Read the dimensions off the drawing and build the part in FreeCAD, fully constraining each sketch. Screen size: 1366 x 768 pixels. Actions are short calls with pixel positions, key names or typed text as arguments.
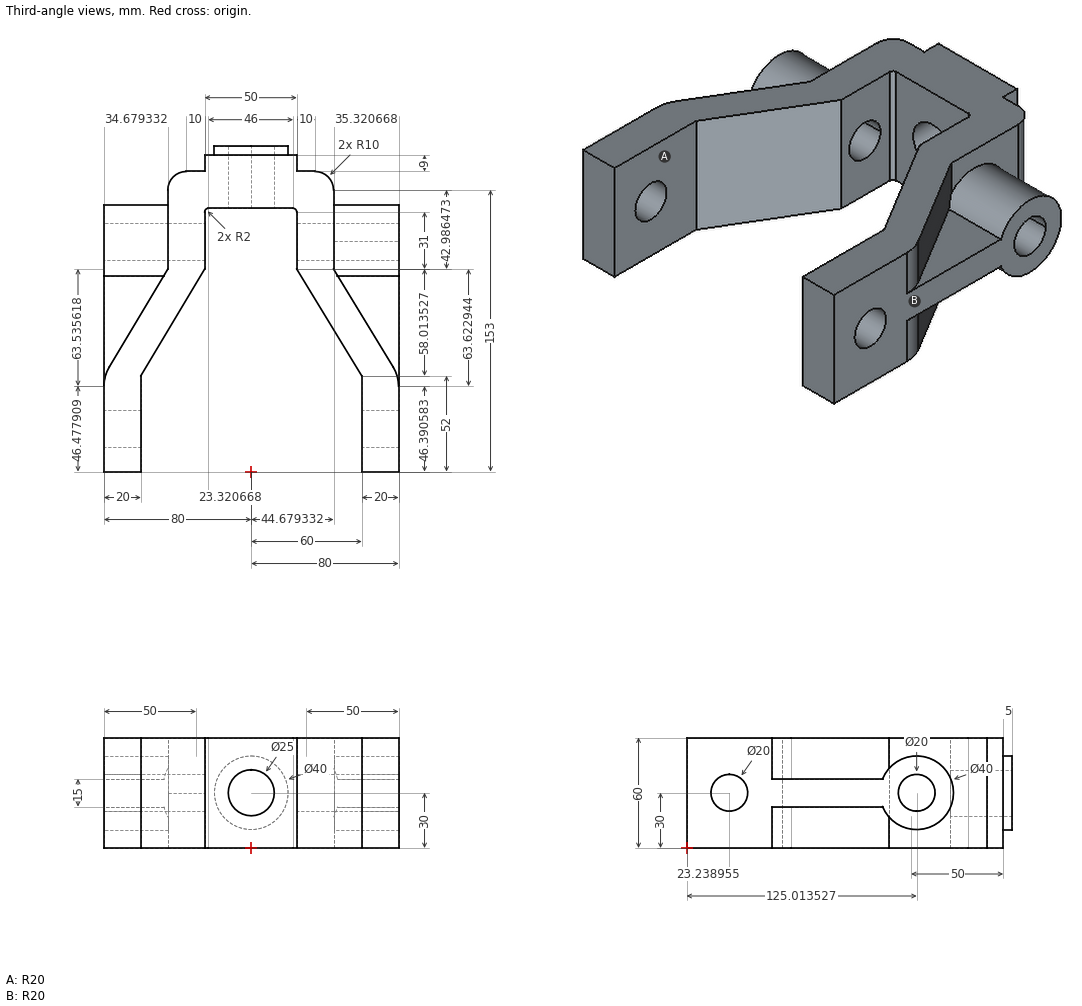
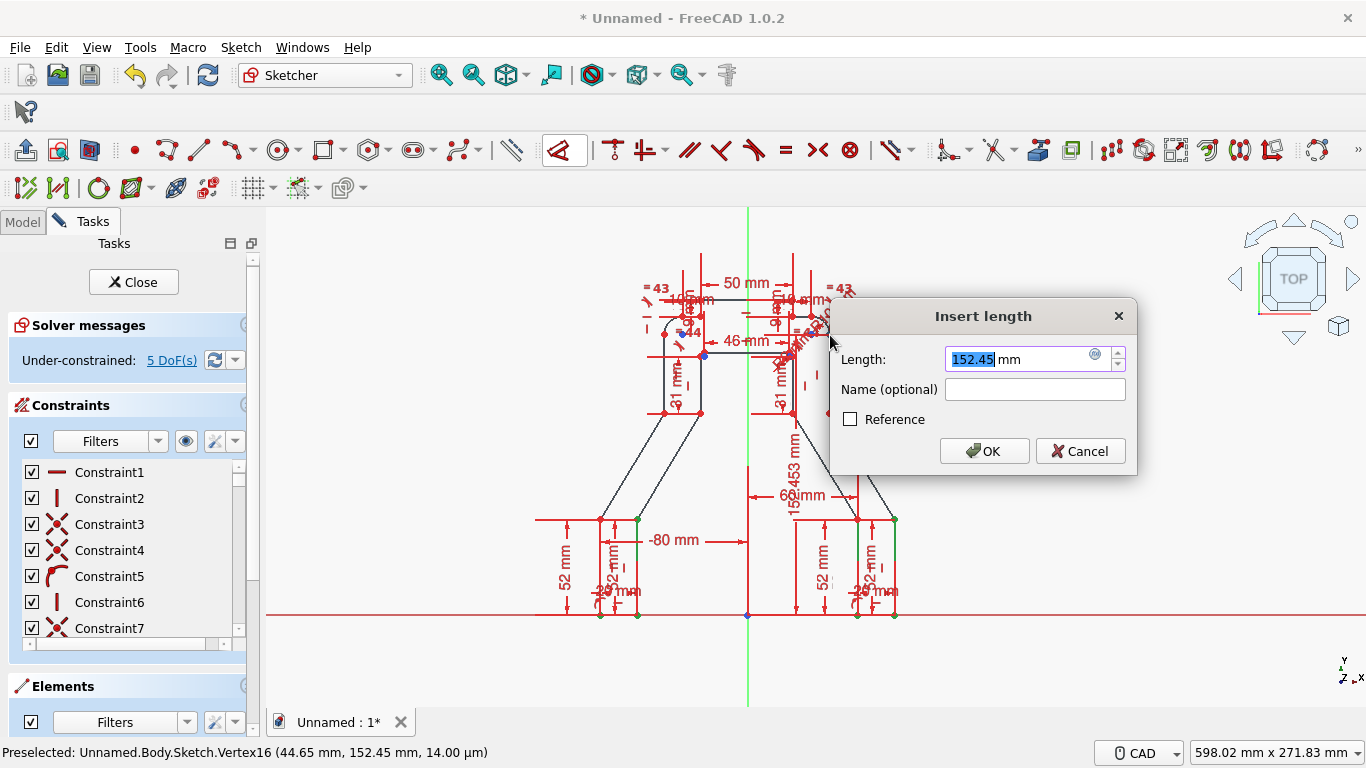
text(153)
key(Return)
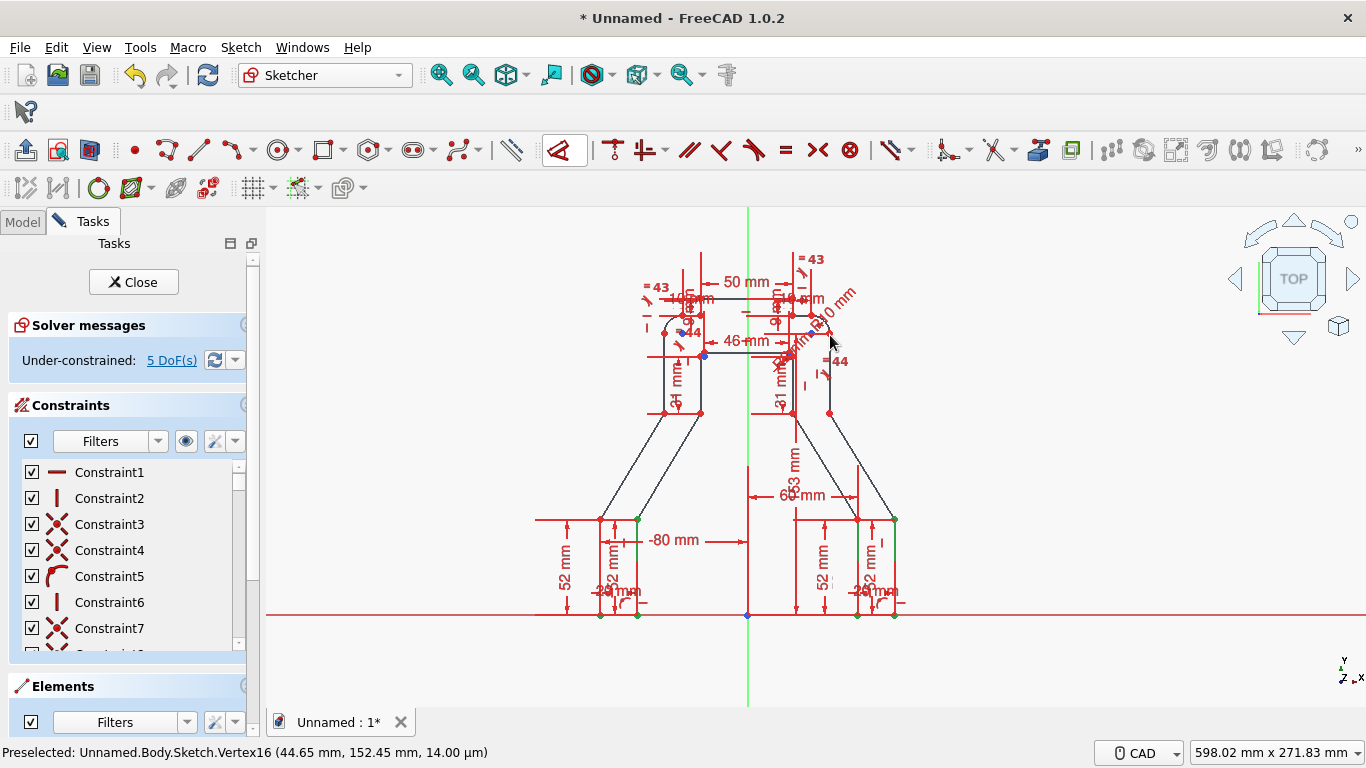
click(830, 390)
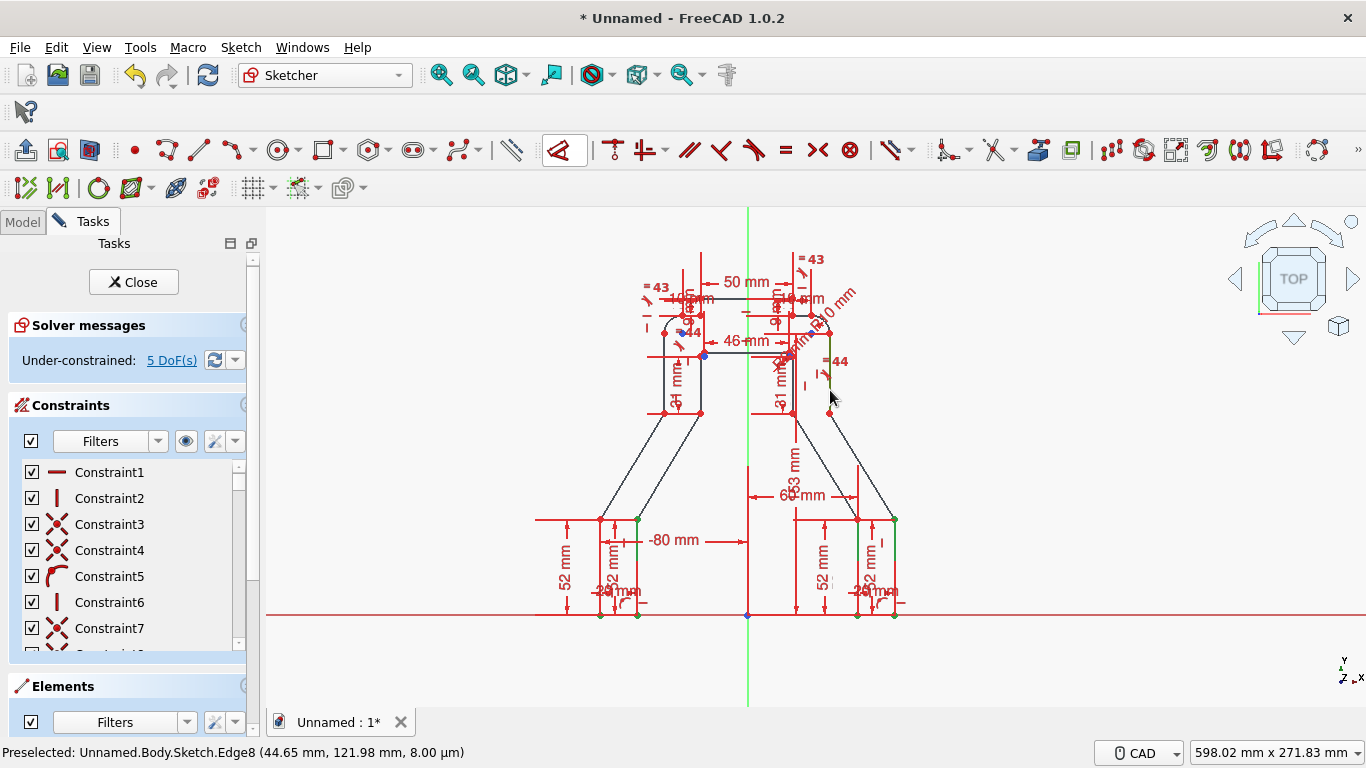
key(i)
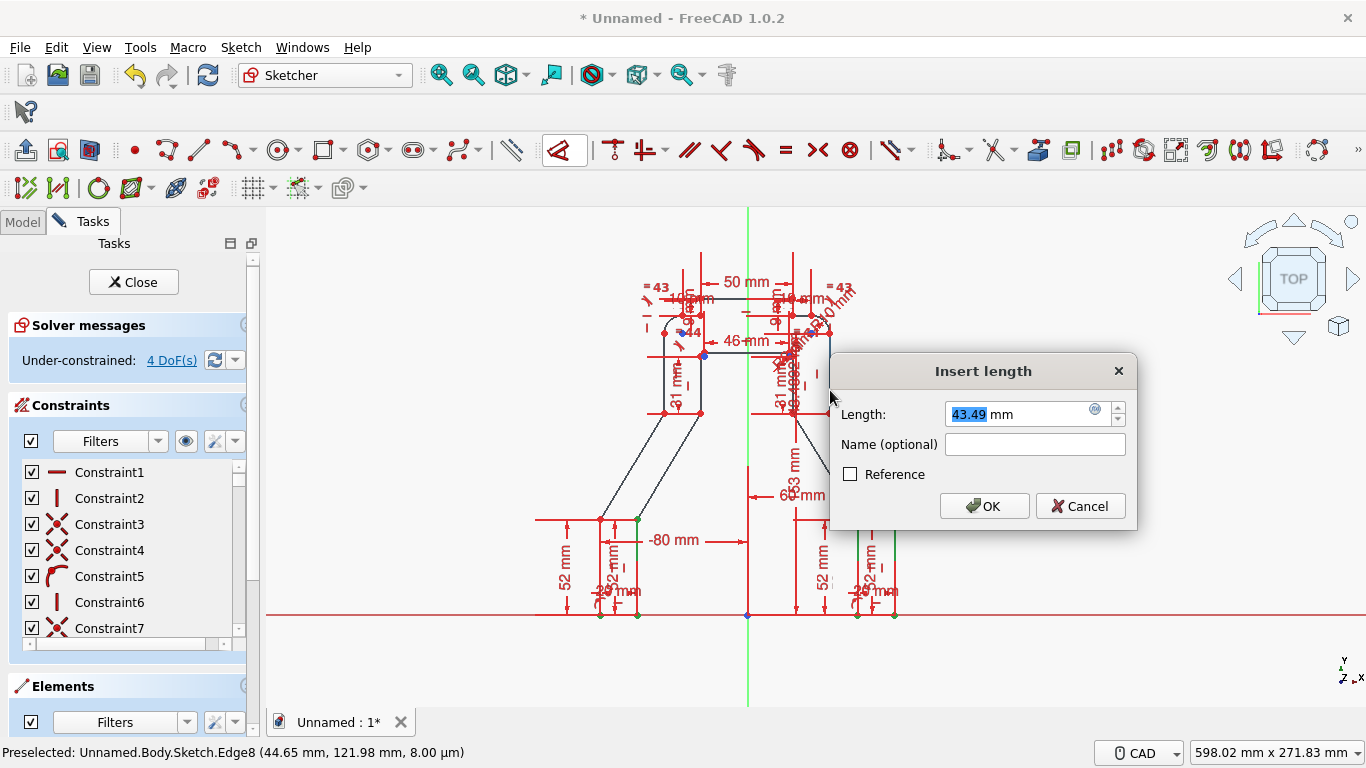
text(42.986473)
key(Return)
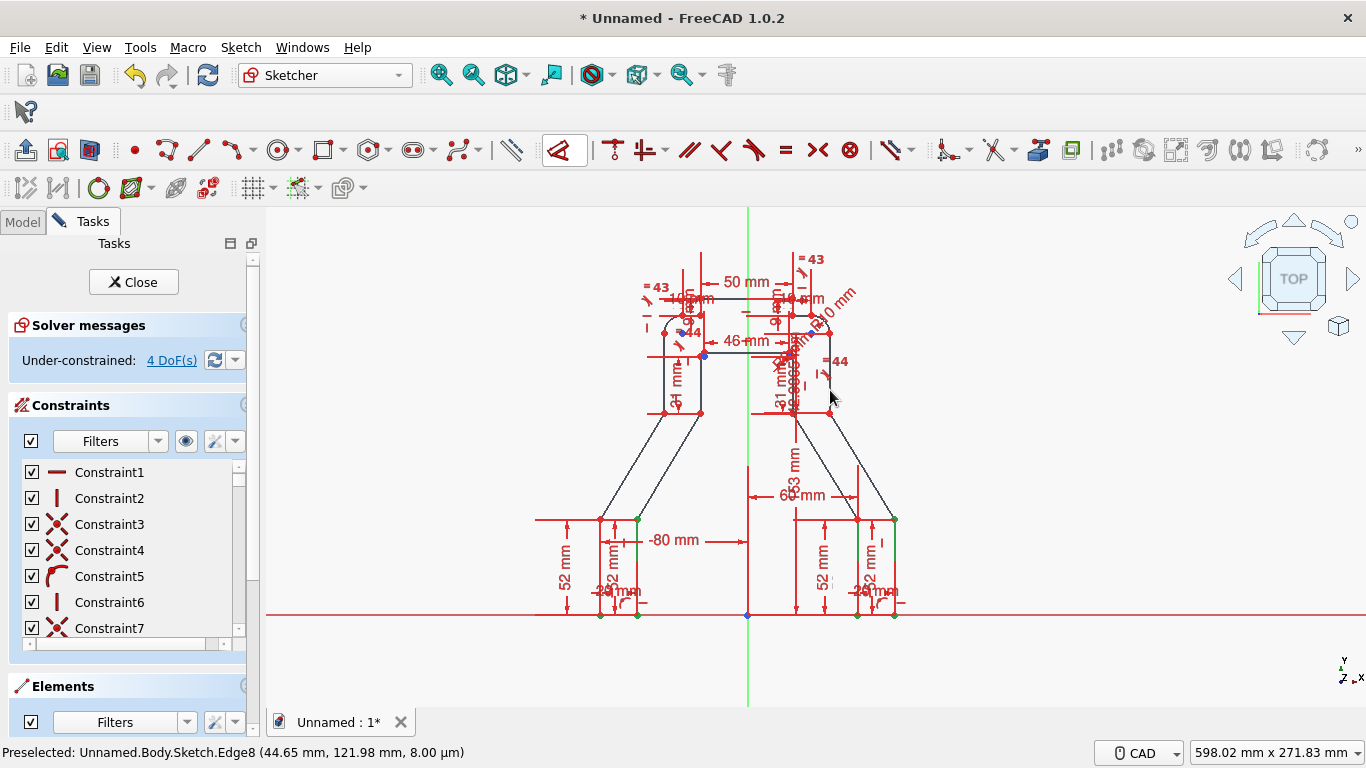
click(664, 358)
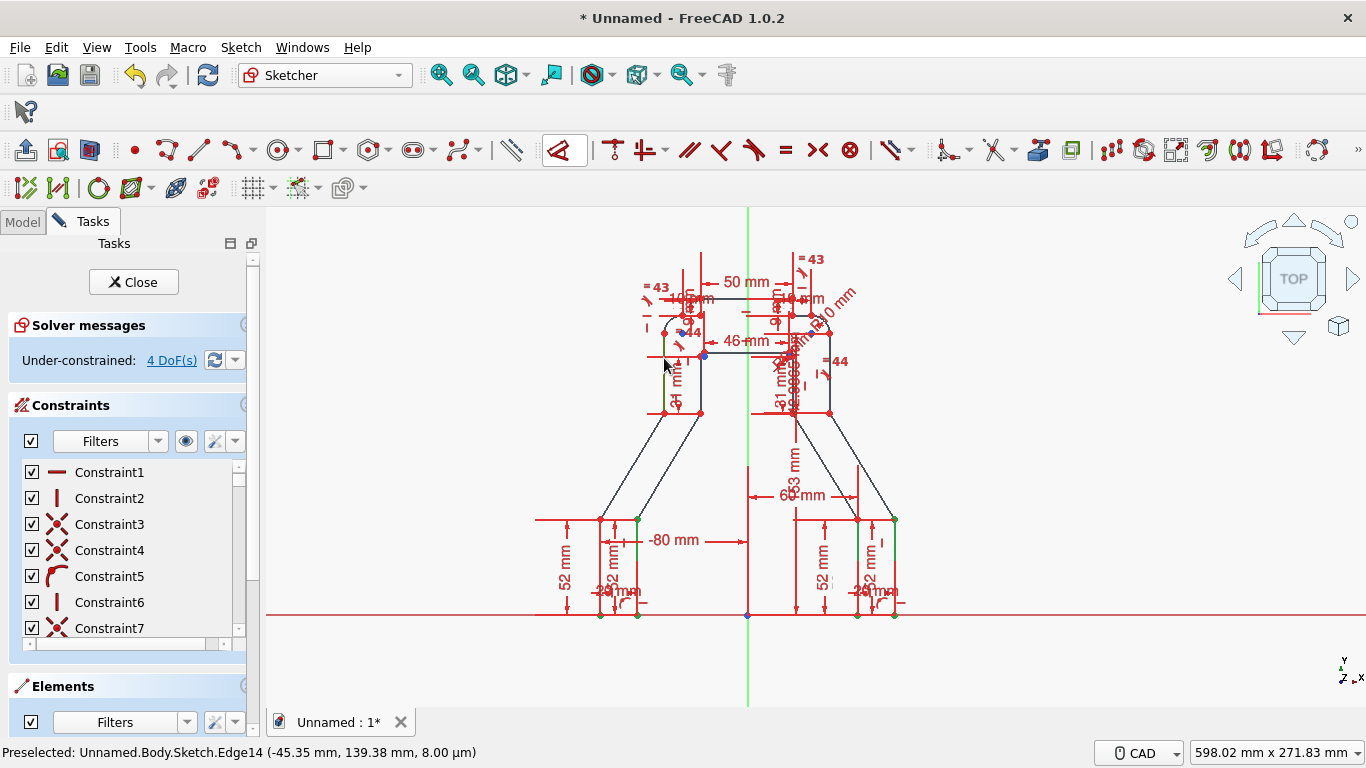
click(582, 150)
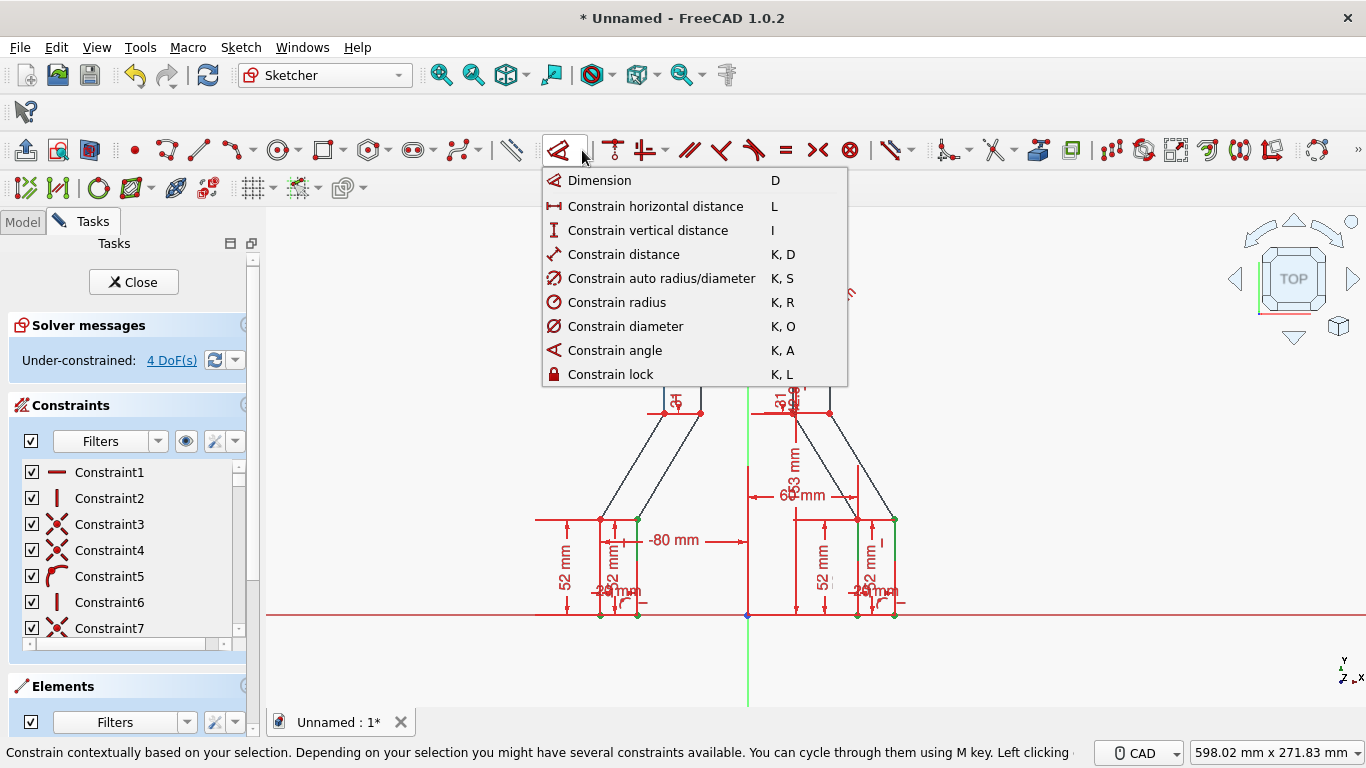
click(695, 230)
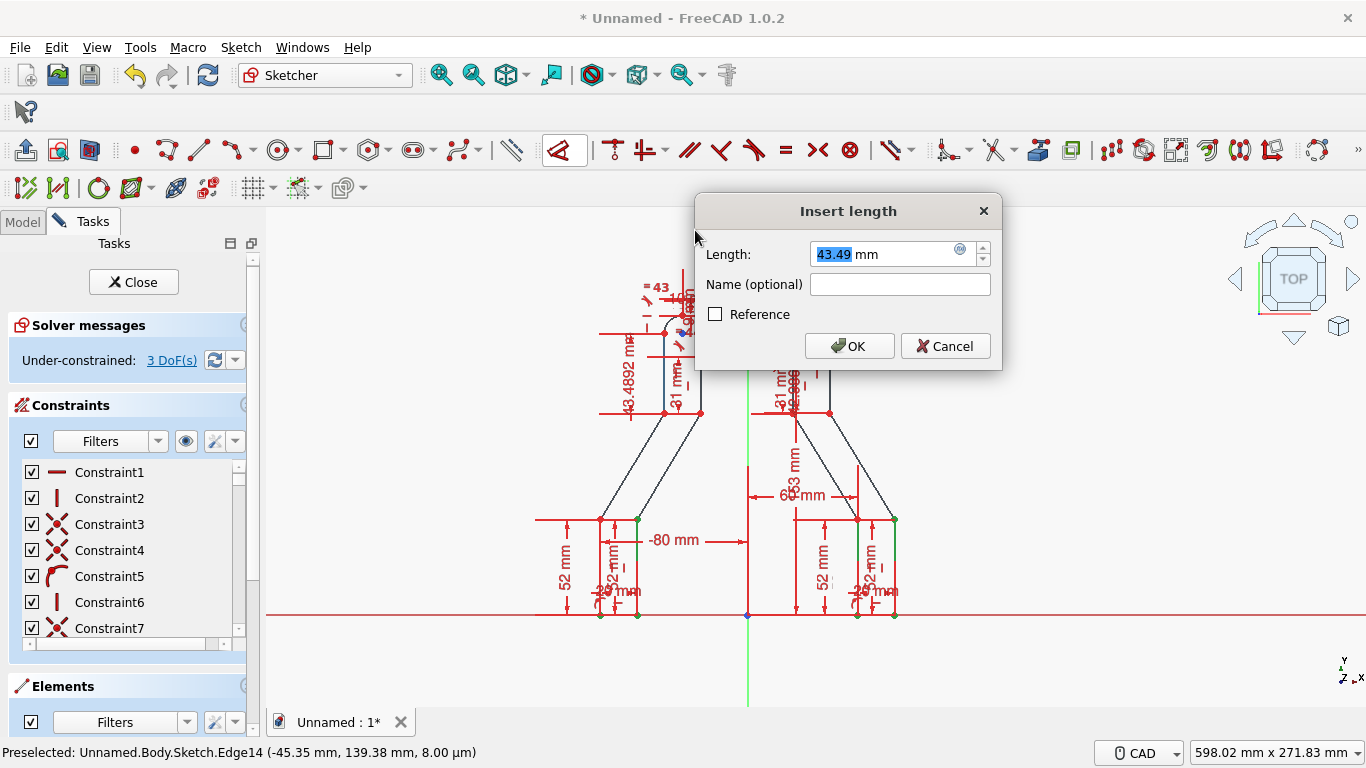
text(42.986473)
key(Return)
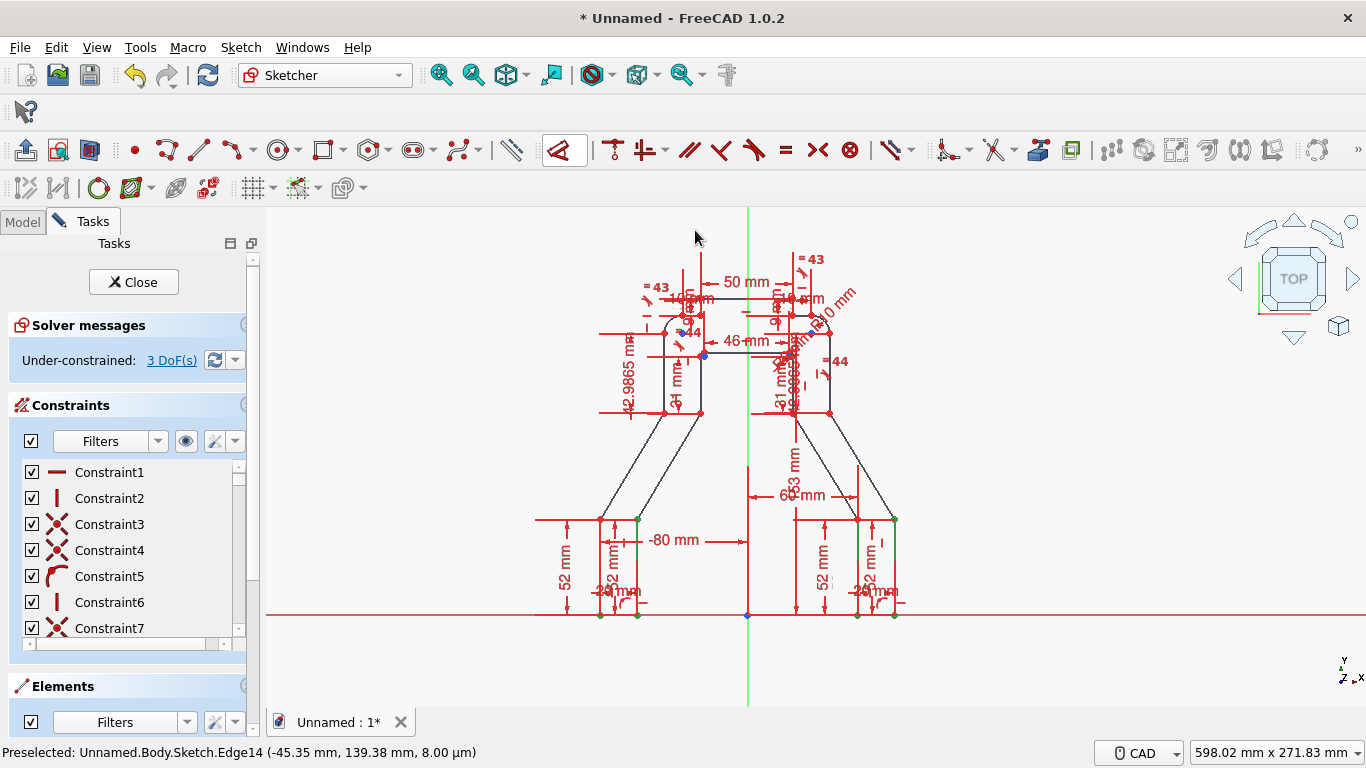
scroll(704, 353, up, 7)